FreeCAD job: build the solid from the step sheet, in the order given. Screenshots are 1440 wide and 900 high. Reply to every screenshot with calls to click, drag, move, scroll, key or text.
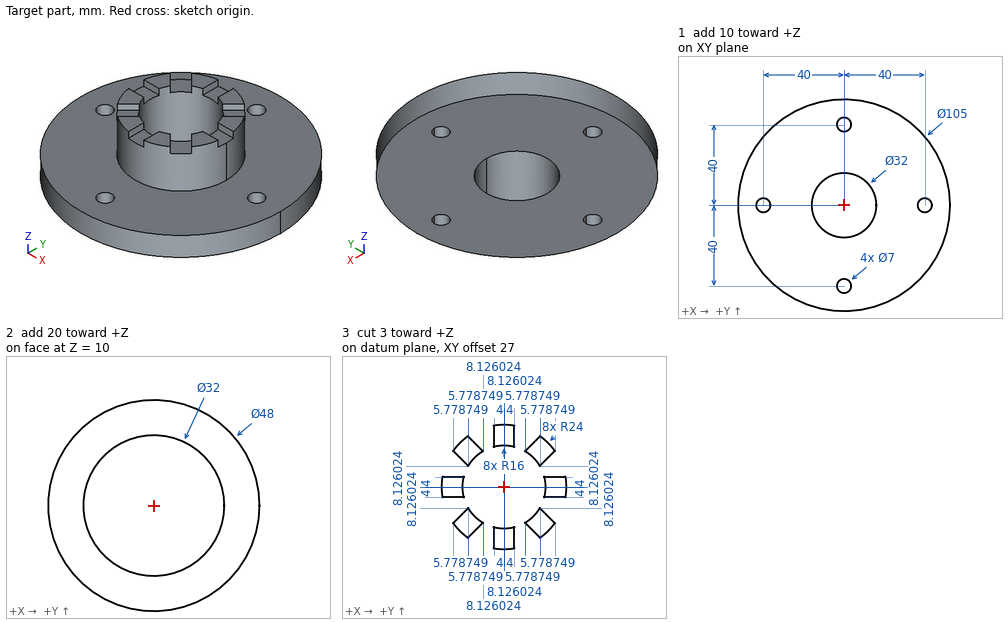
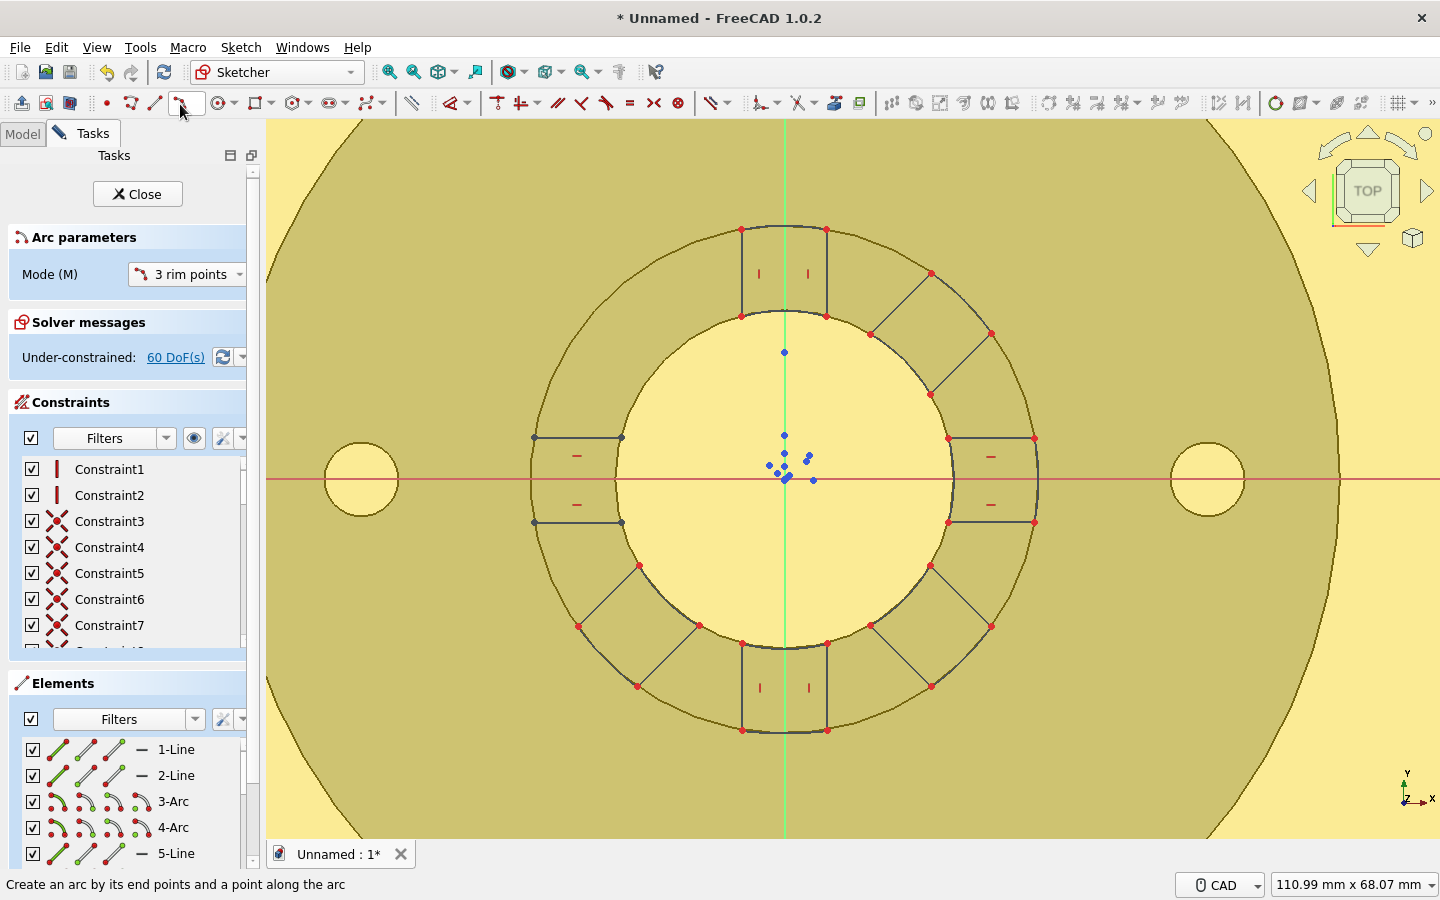
click(621, 523)
click(621, 438)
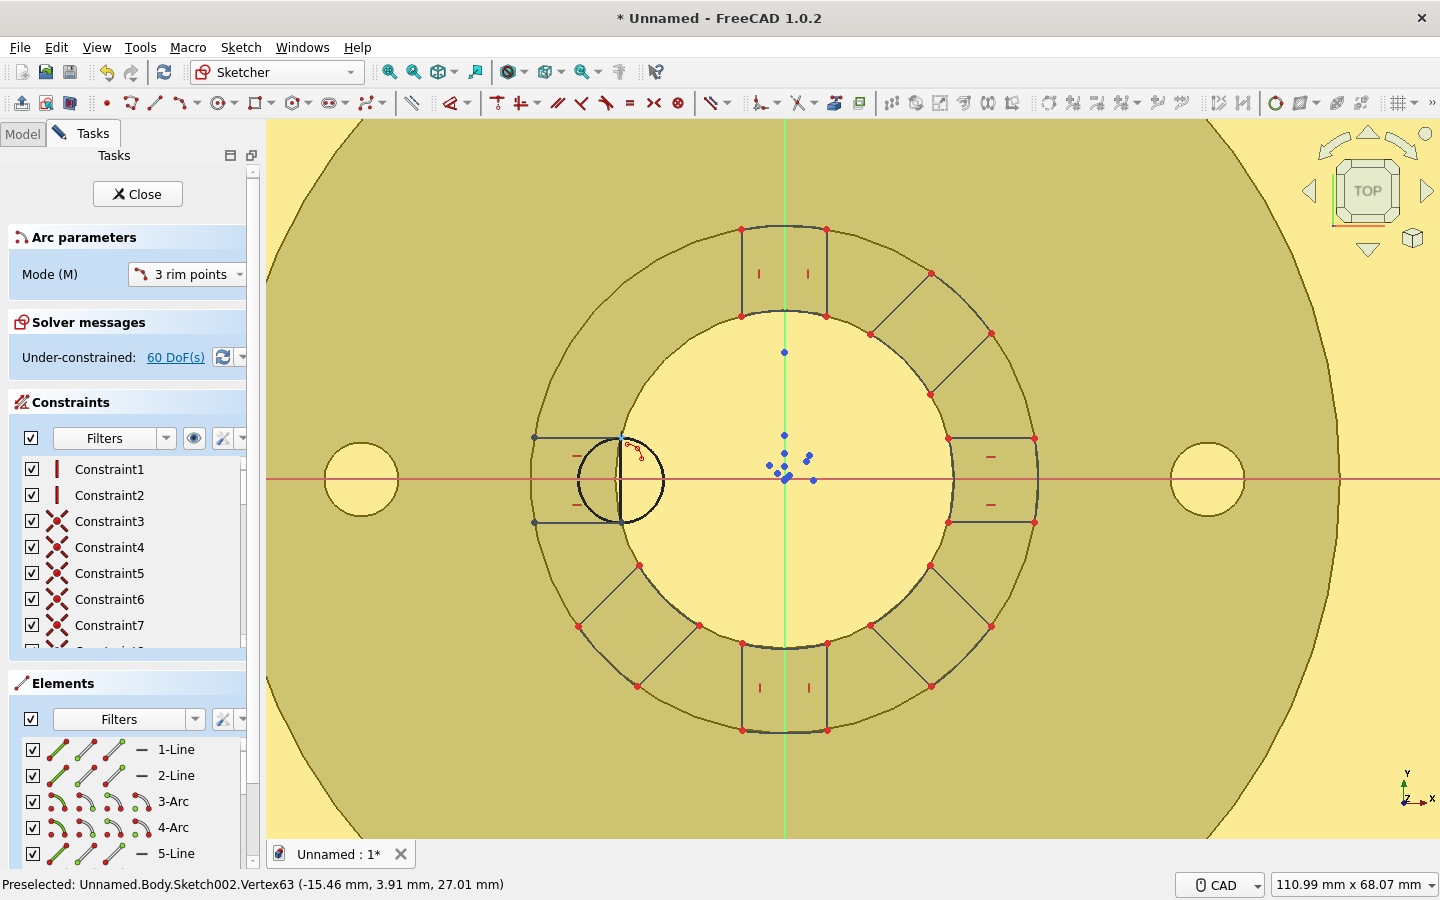
scroll(616, 471, up, 6)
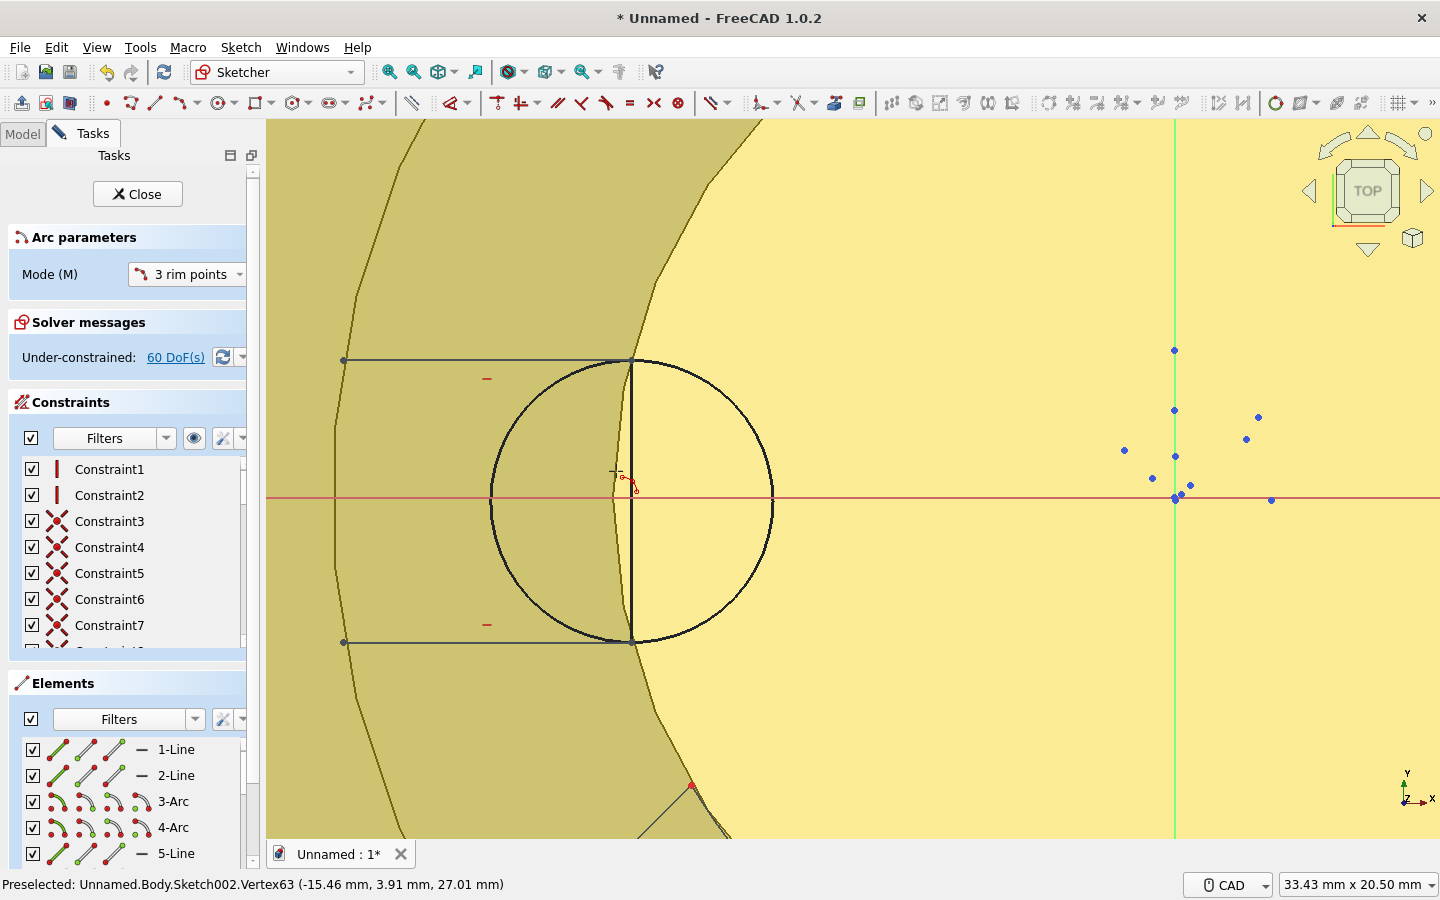
click(614, 469)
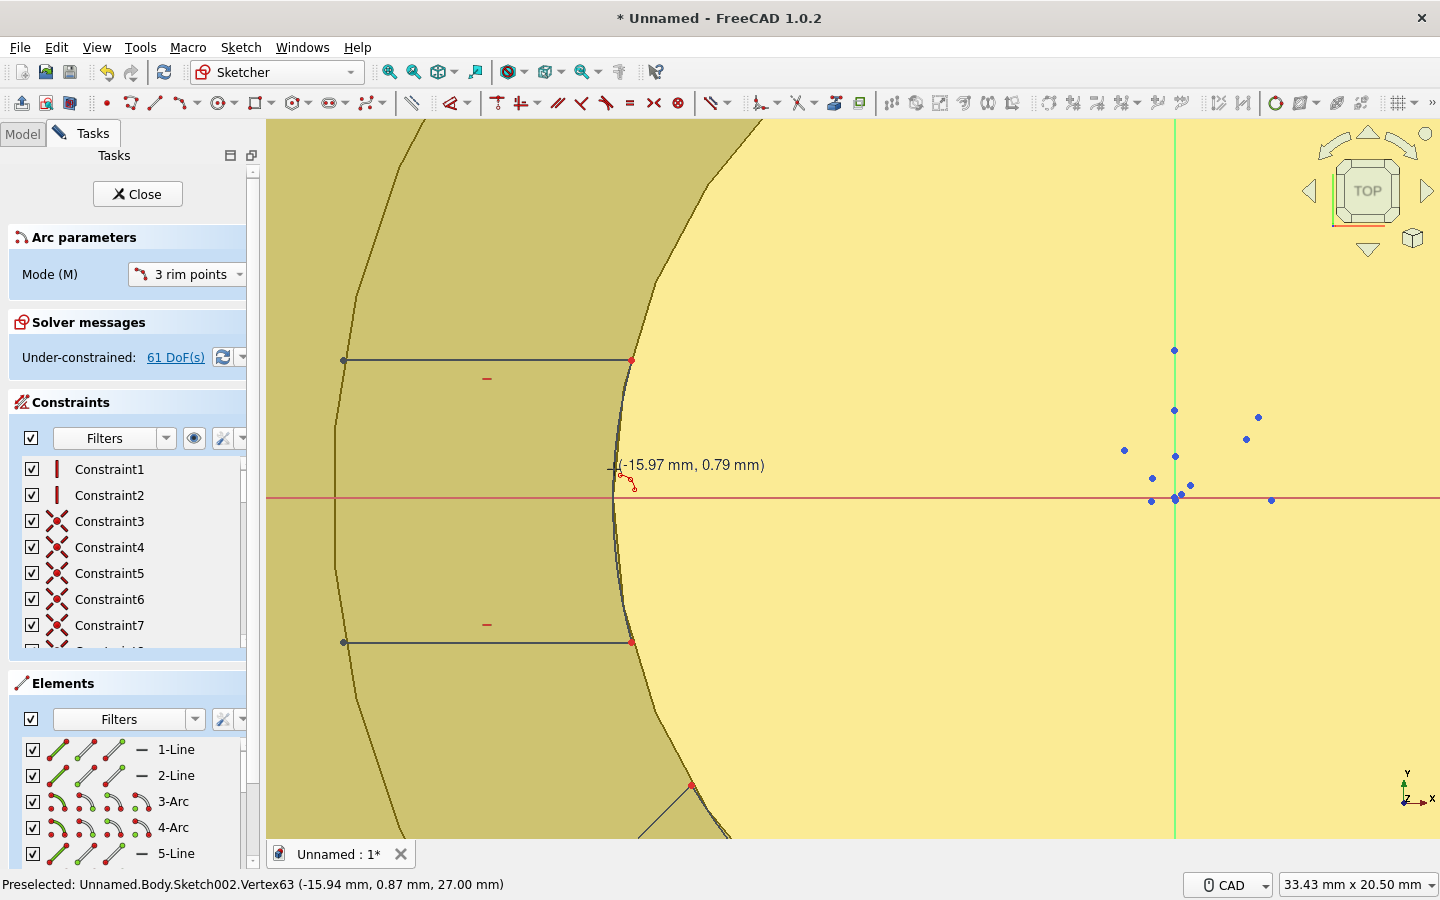
click(343, 360)
click(343, 643)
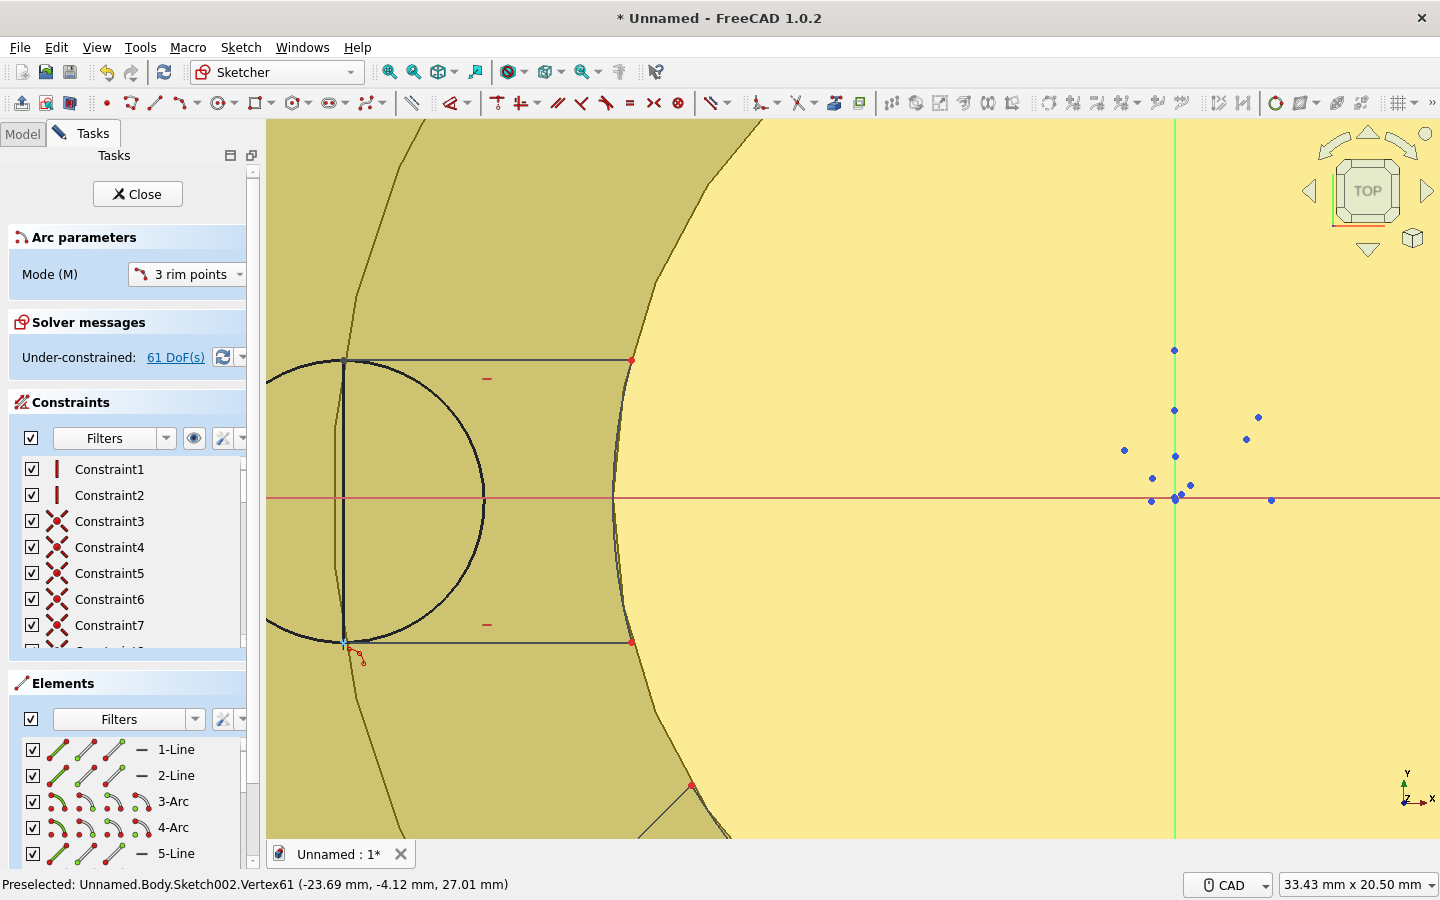
scroll(332, 469, up, 2)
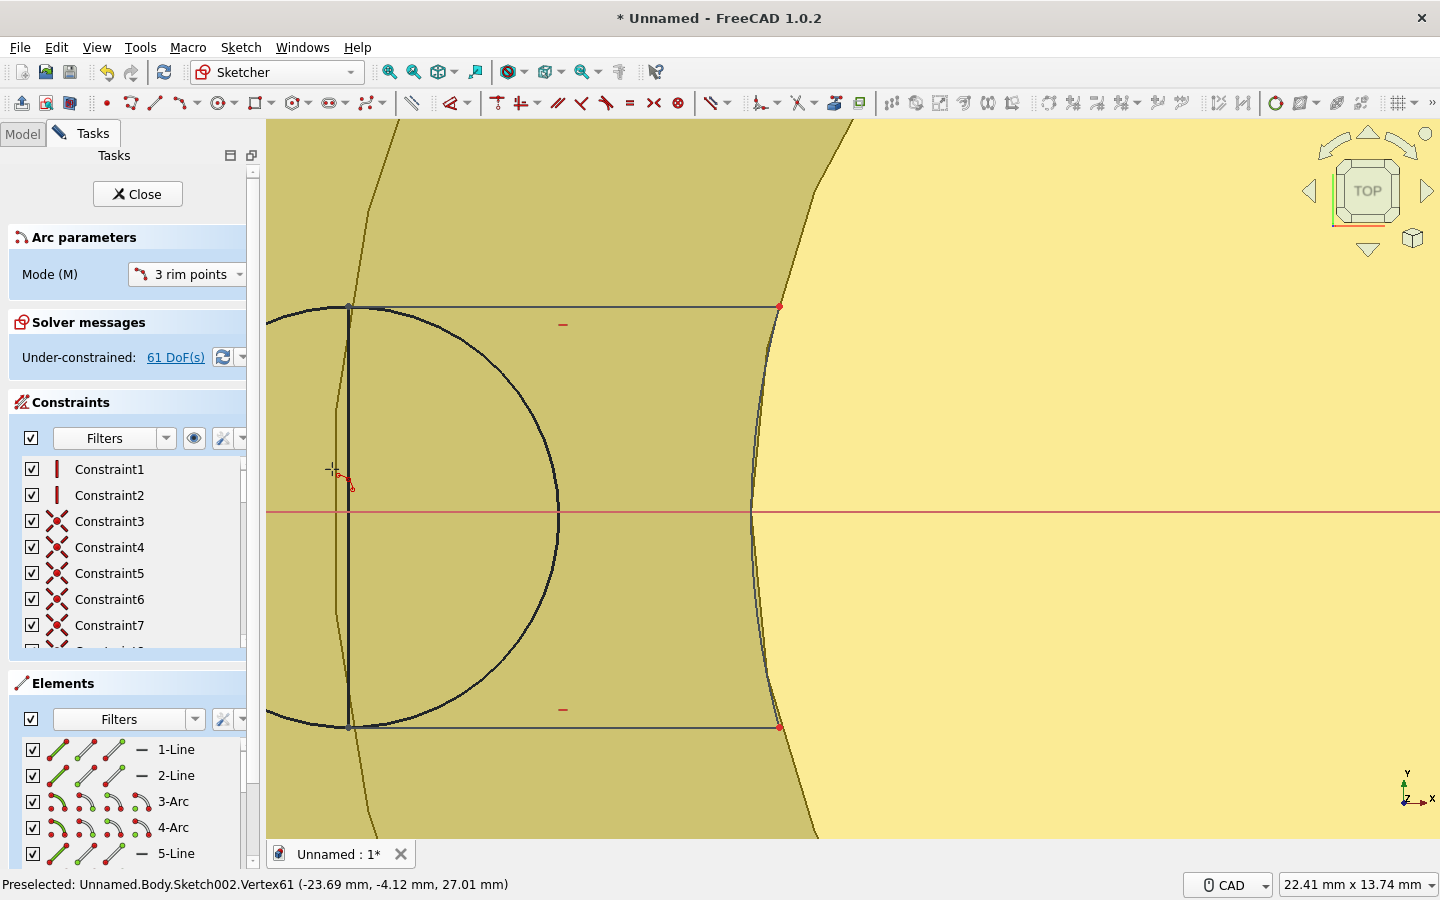
click(333, 469)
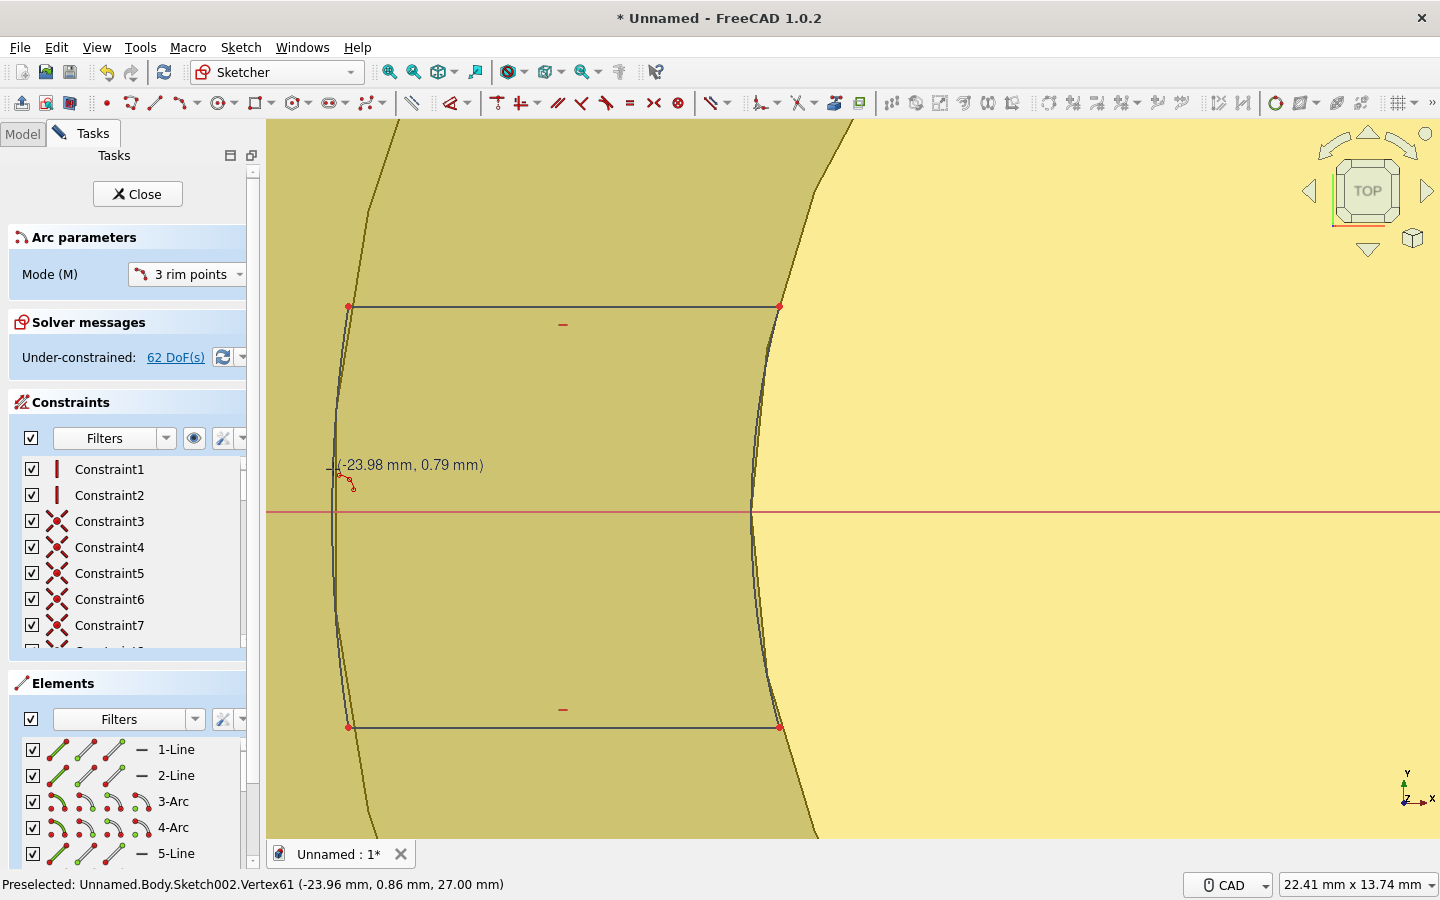
click(156, 104)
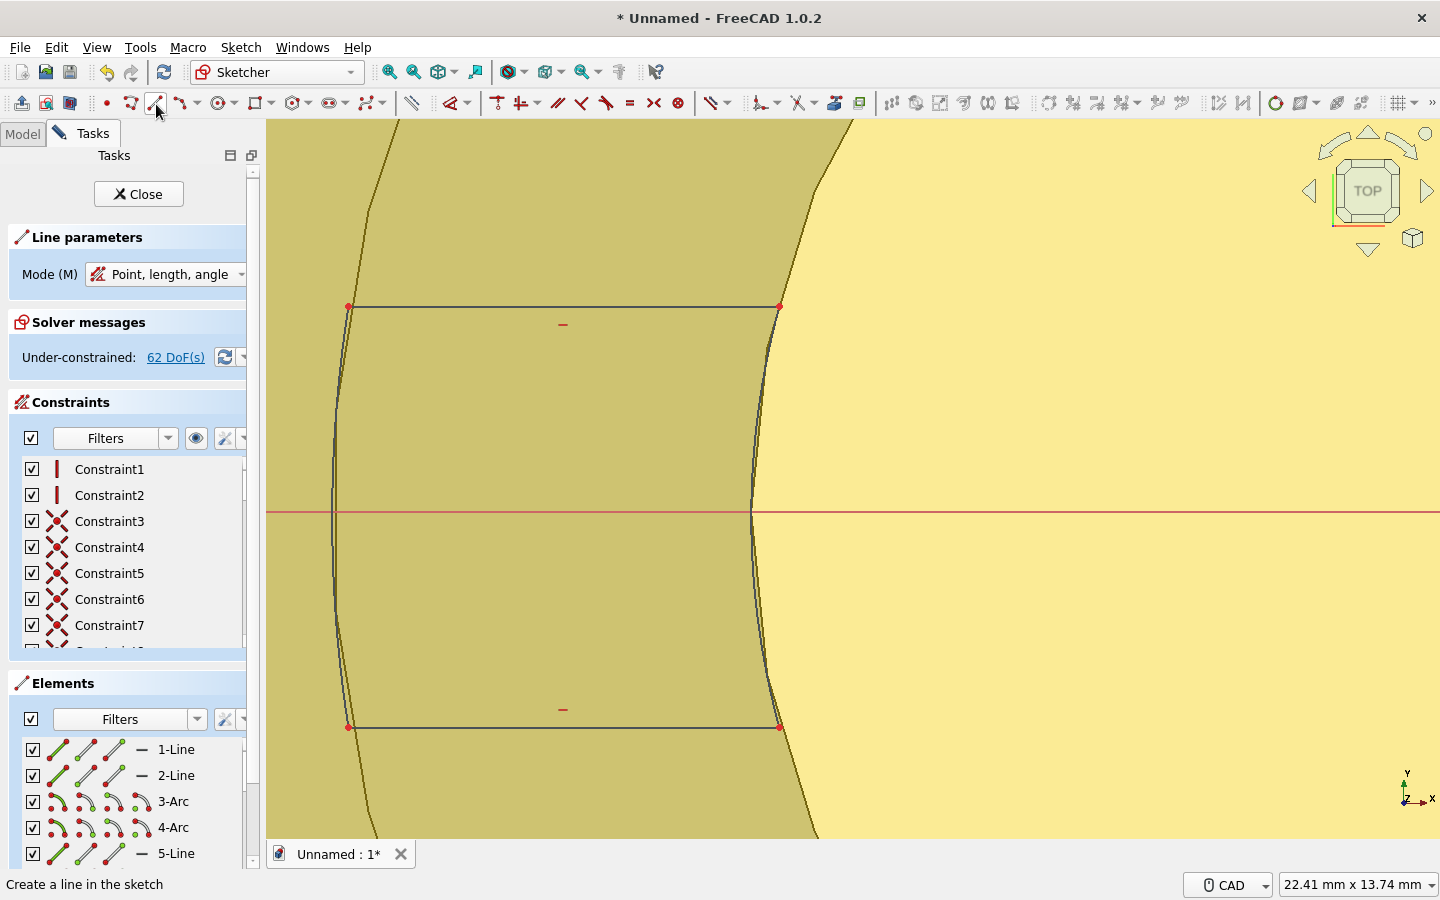
scroll(581, 471, down, 8)